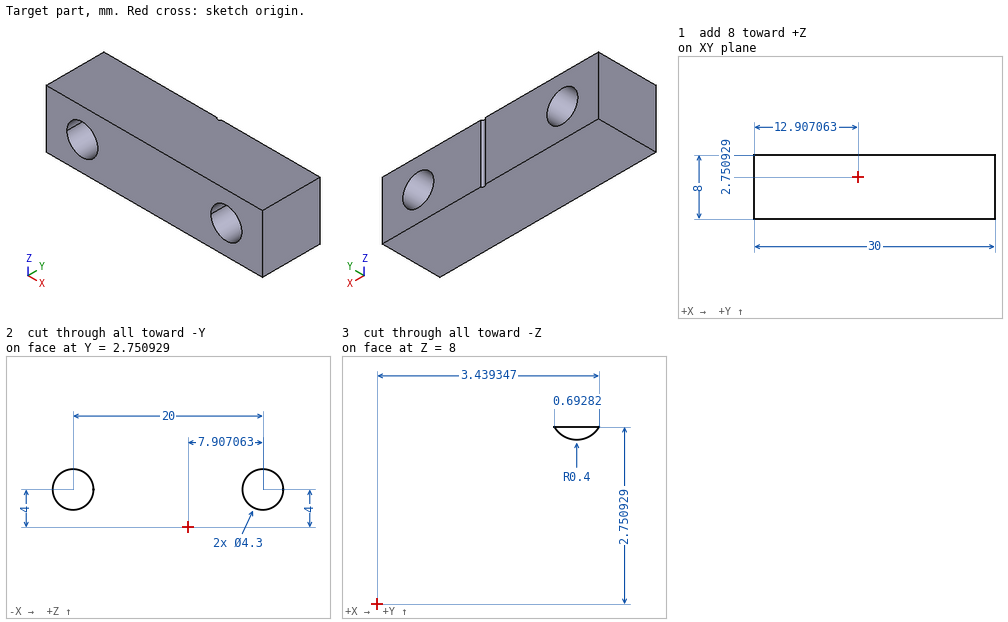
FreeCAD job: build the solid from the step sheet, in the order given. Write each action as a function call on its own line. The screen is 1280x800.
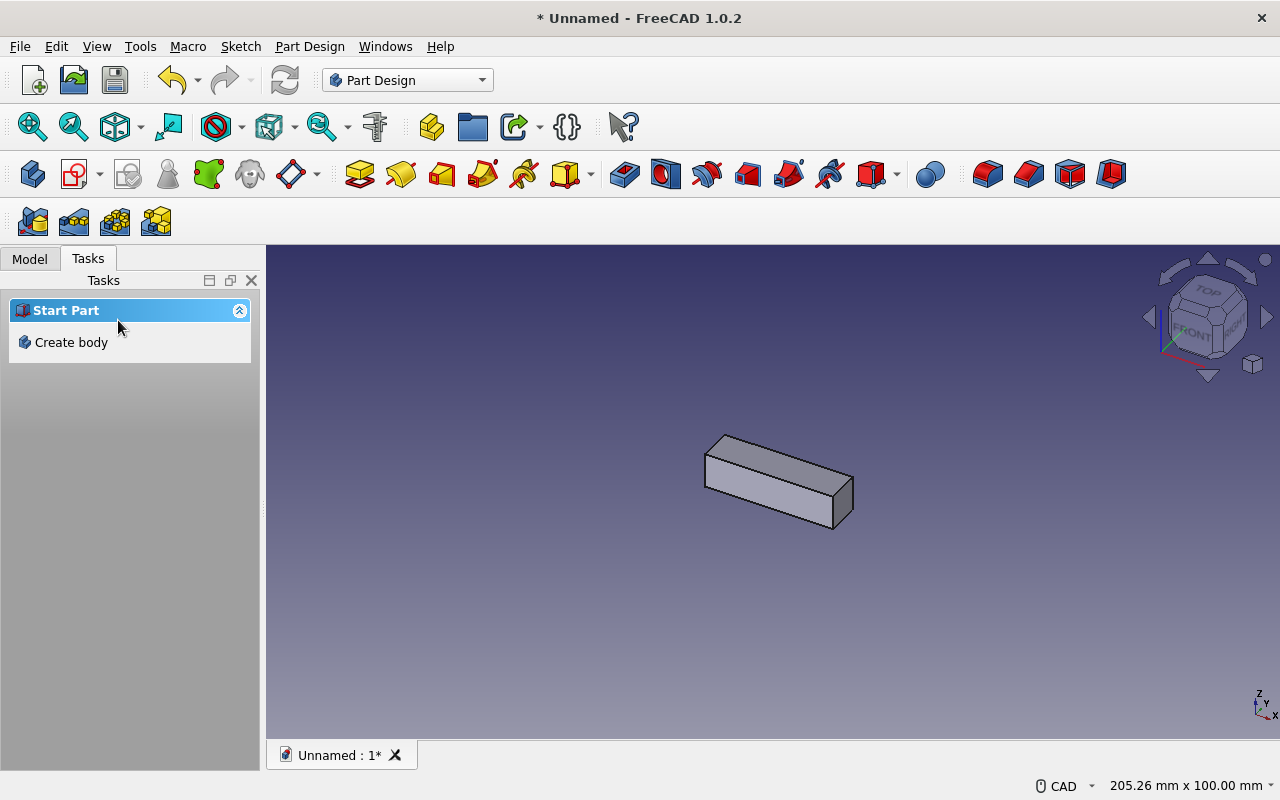
click(33, 128)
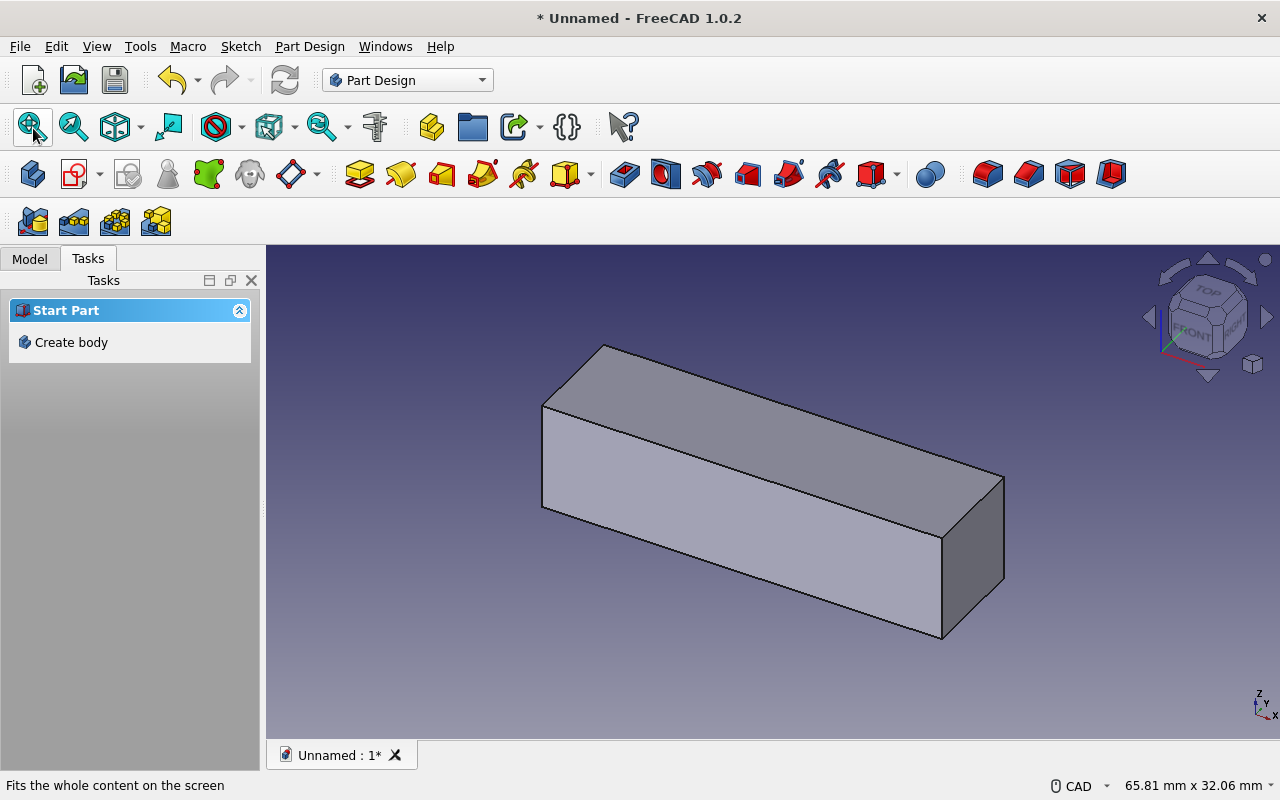
key(4)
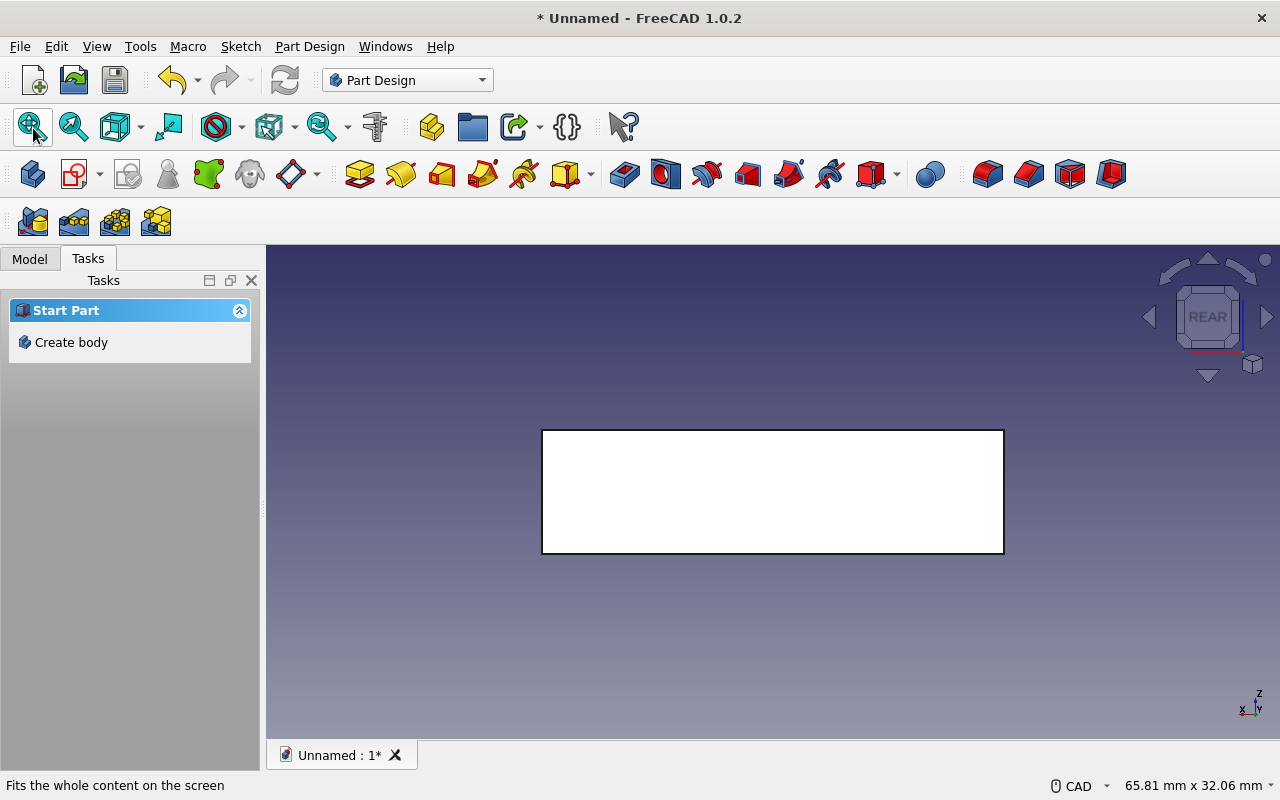
click(641, 491)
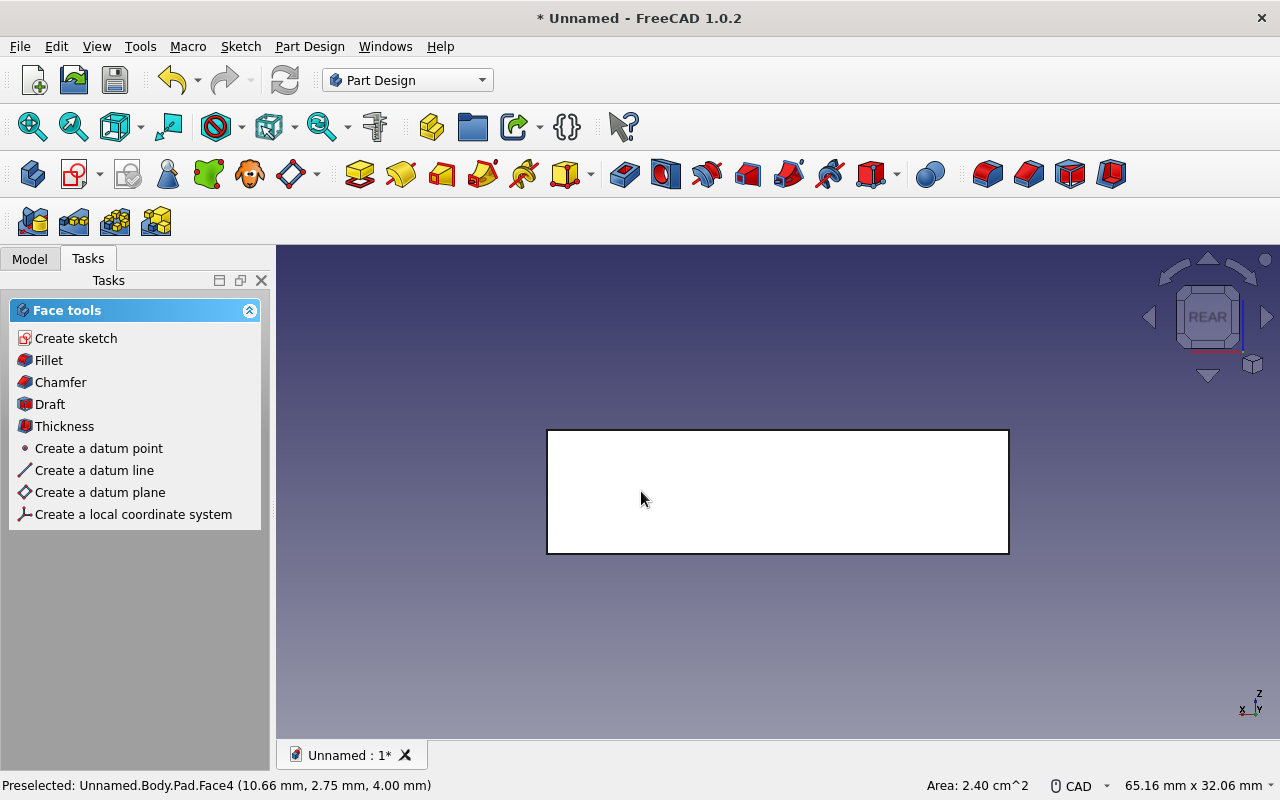
click(74, 174)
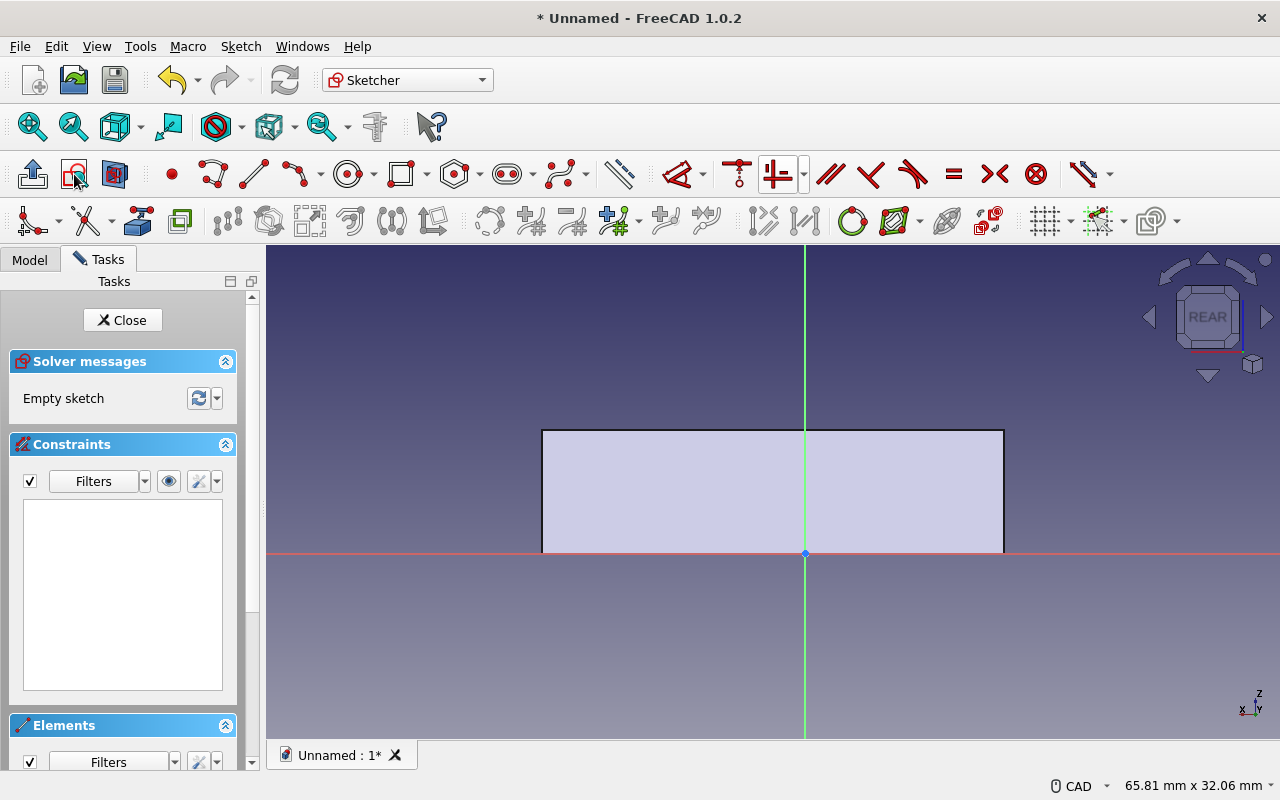
scroll(912, 535, up, 2)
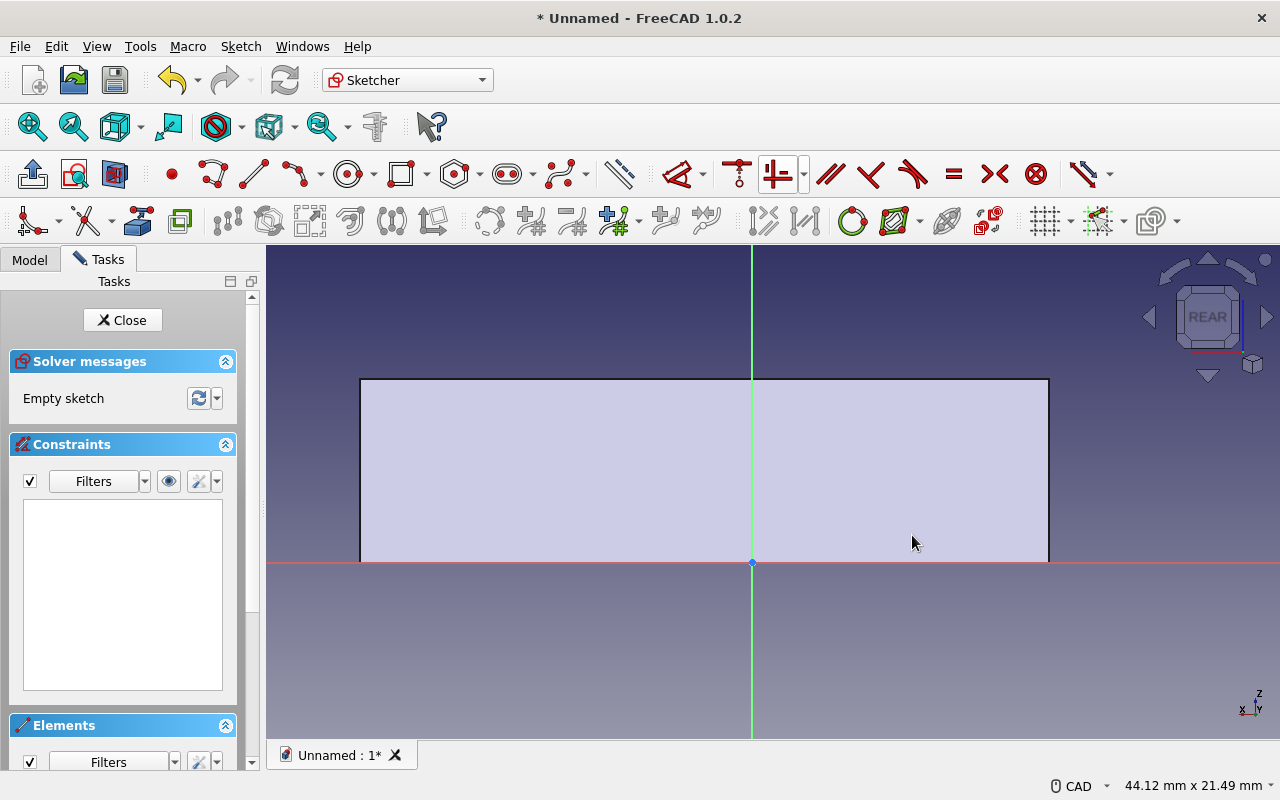
key(g)
key(c)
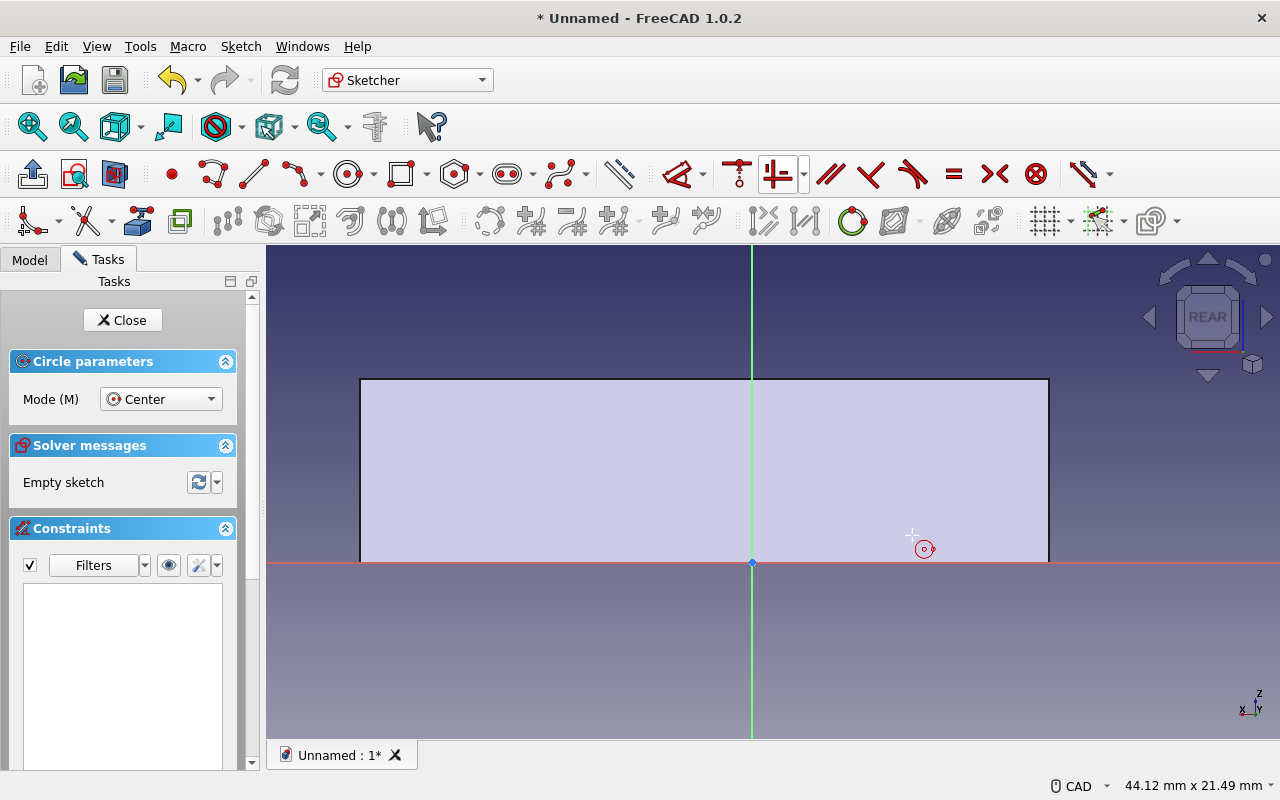
click(934, 471)
click(969, 436)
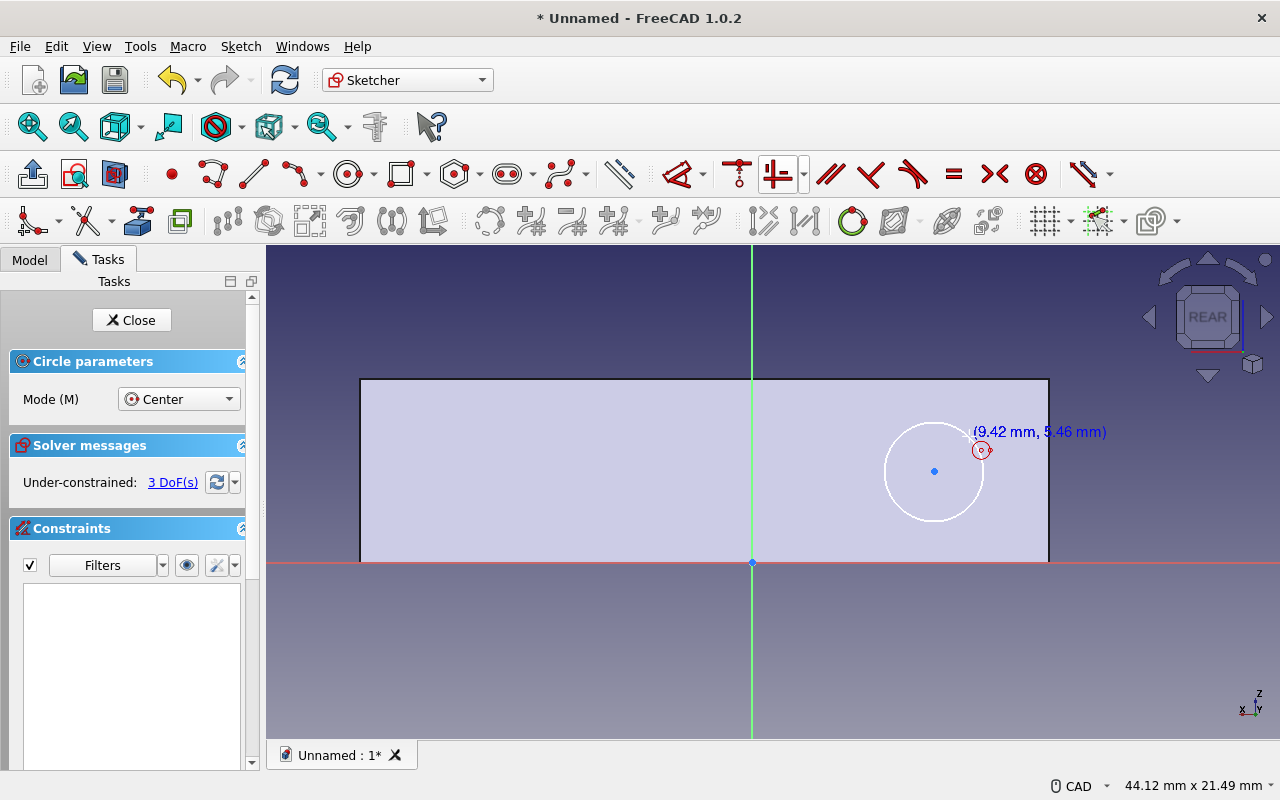
click(474, 471)
click(509, 436)
key(Escape)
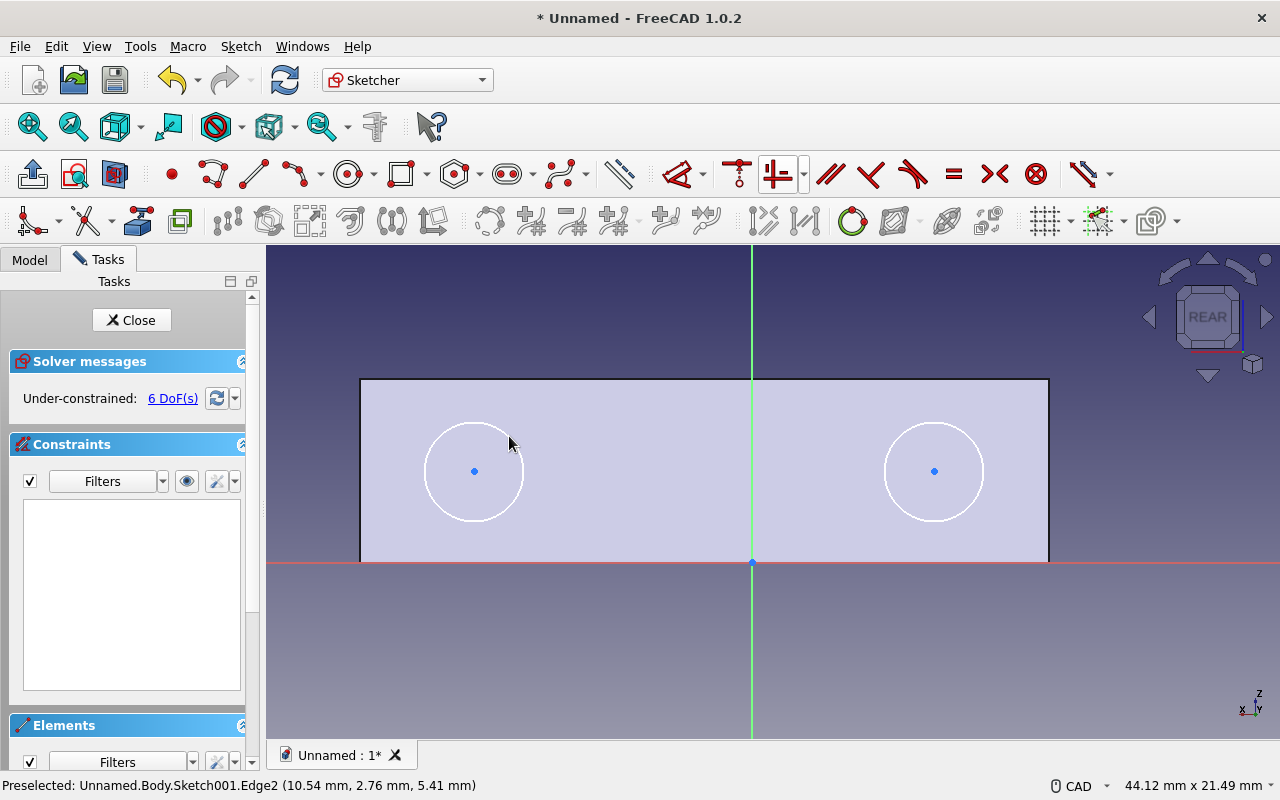
click(969, 437)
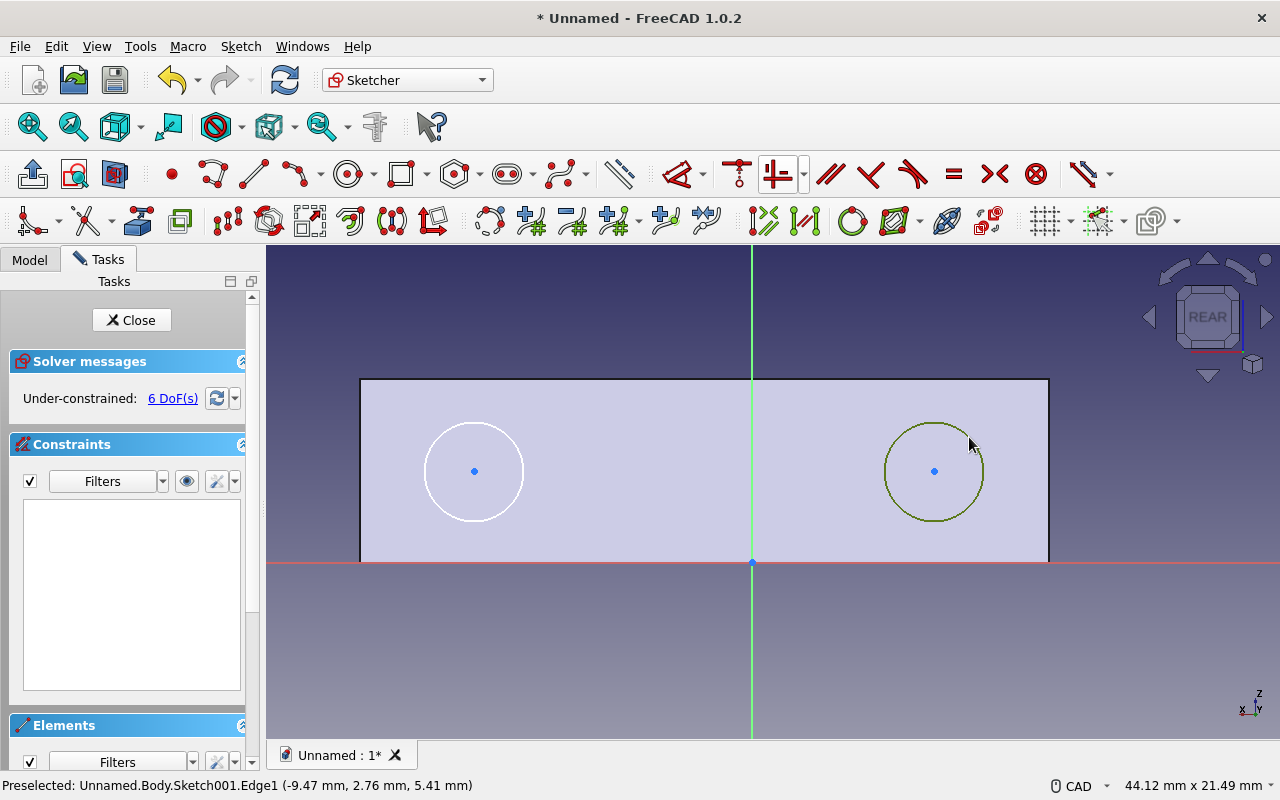
click(509, 437)